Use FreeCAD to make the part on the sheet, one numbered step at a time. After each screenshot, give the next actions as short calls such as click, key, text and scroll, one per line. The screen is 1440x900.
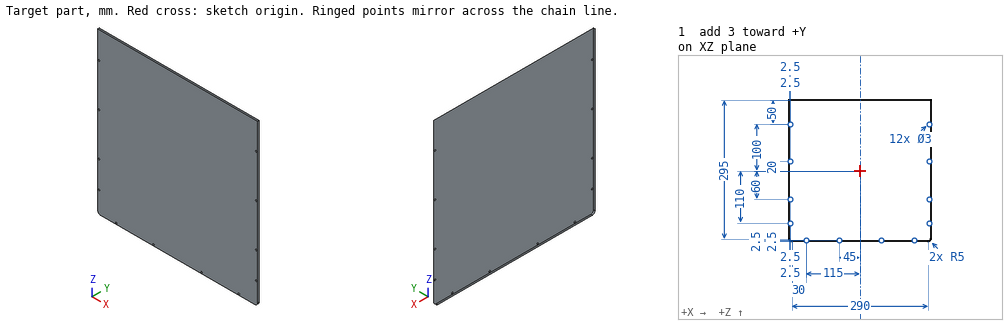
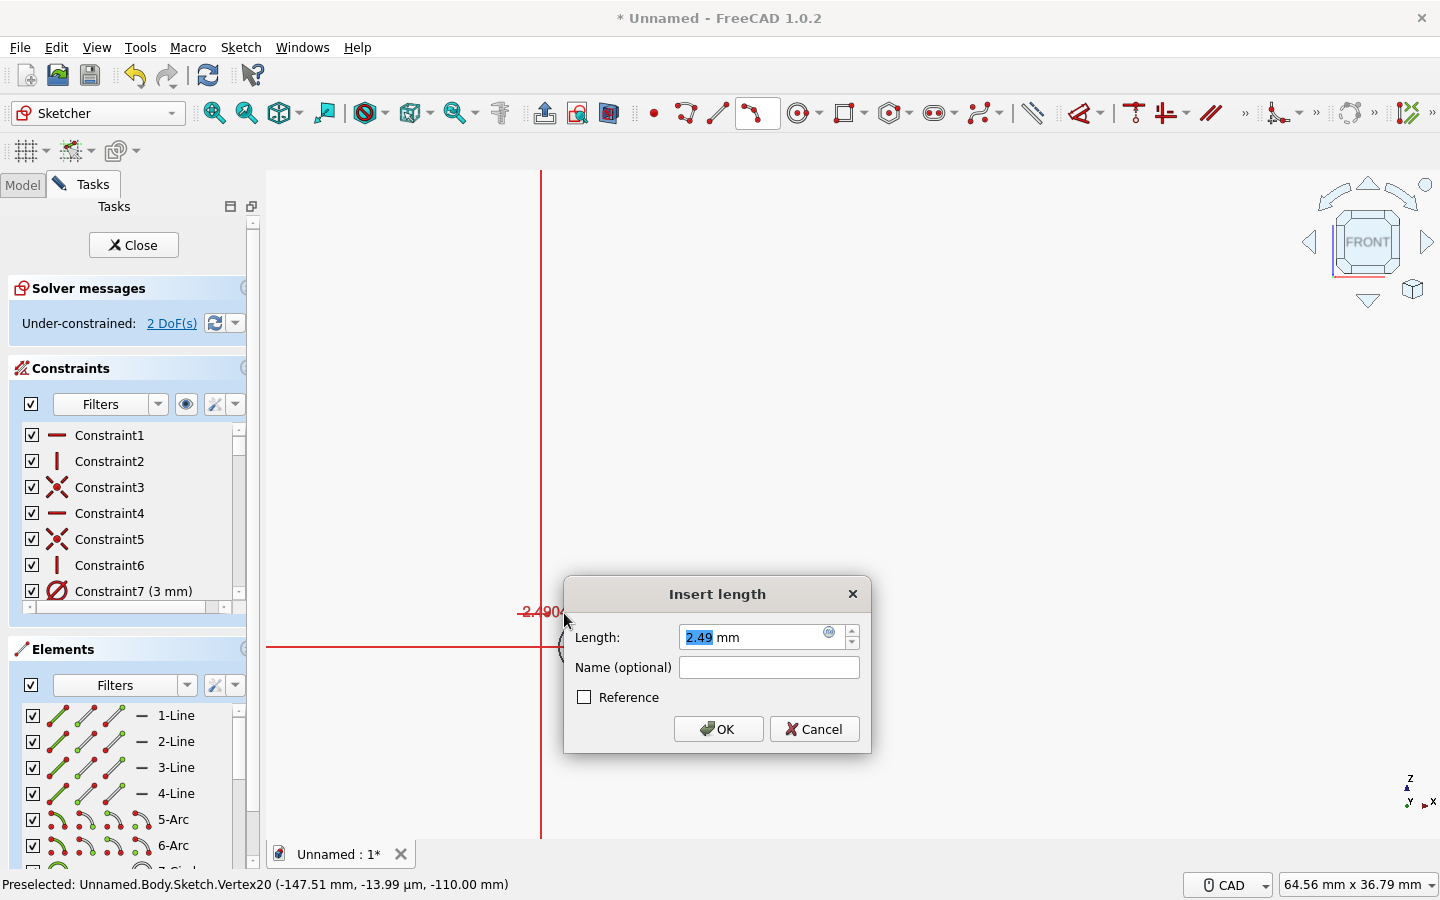
text(2.5)
key(Return)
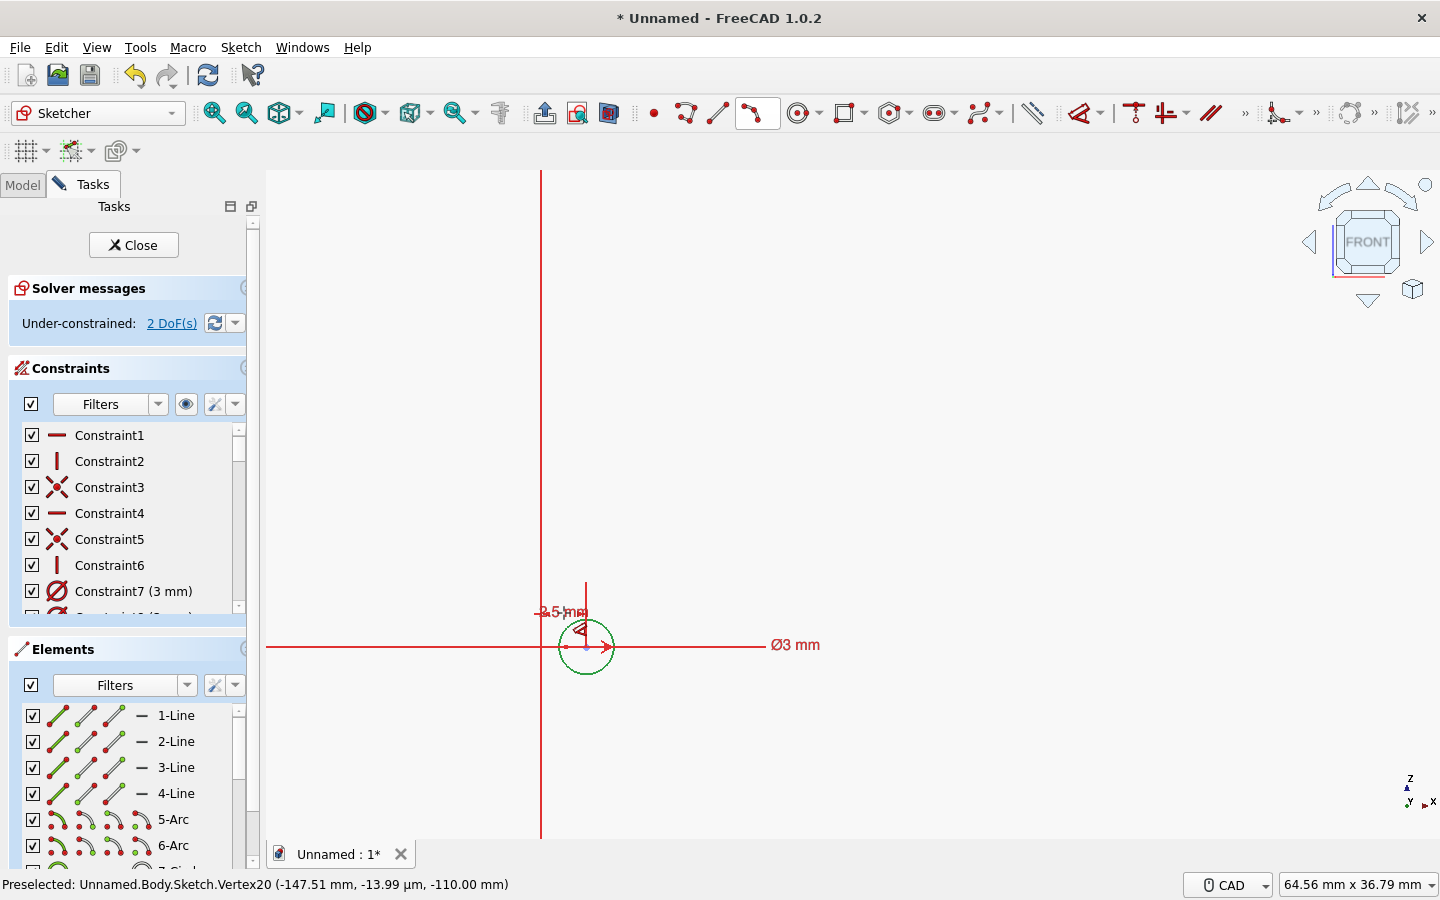
scroll(585, 654, down, 13)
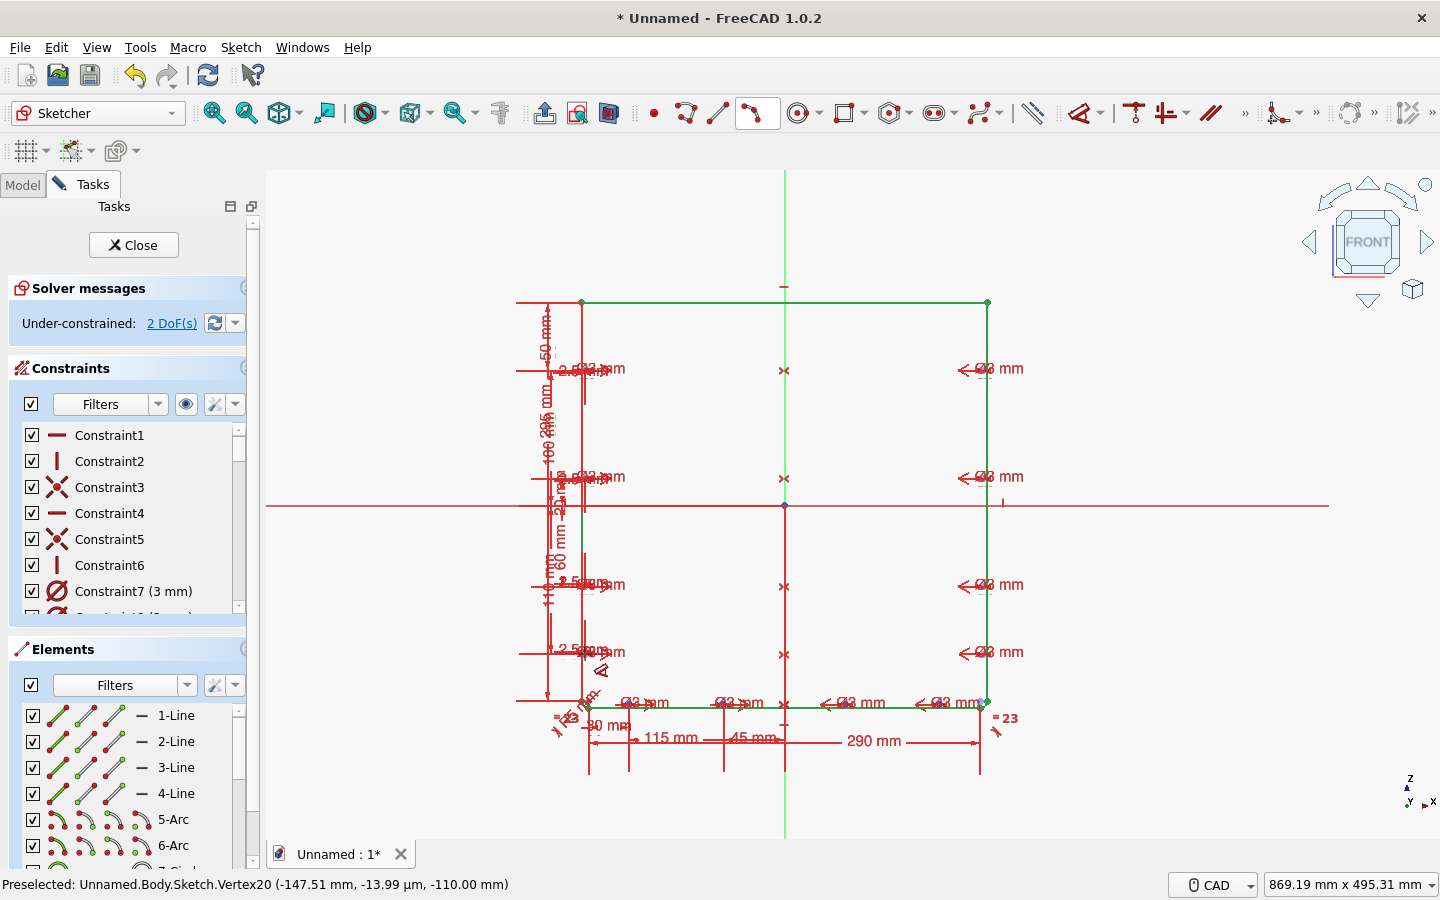
scroll(589, 708, up, 13)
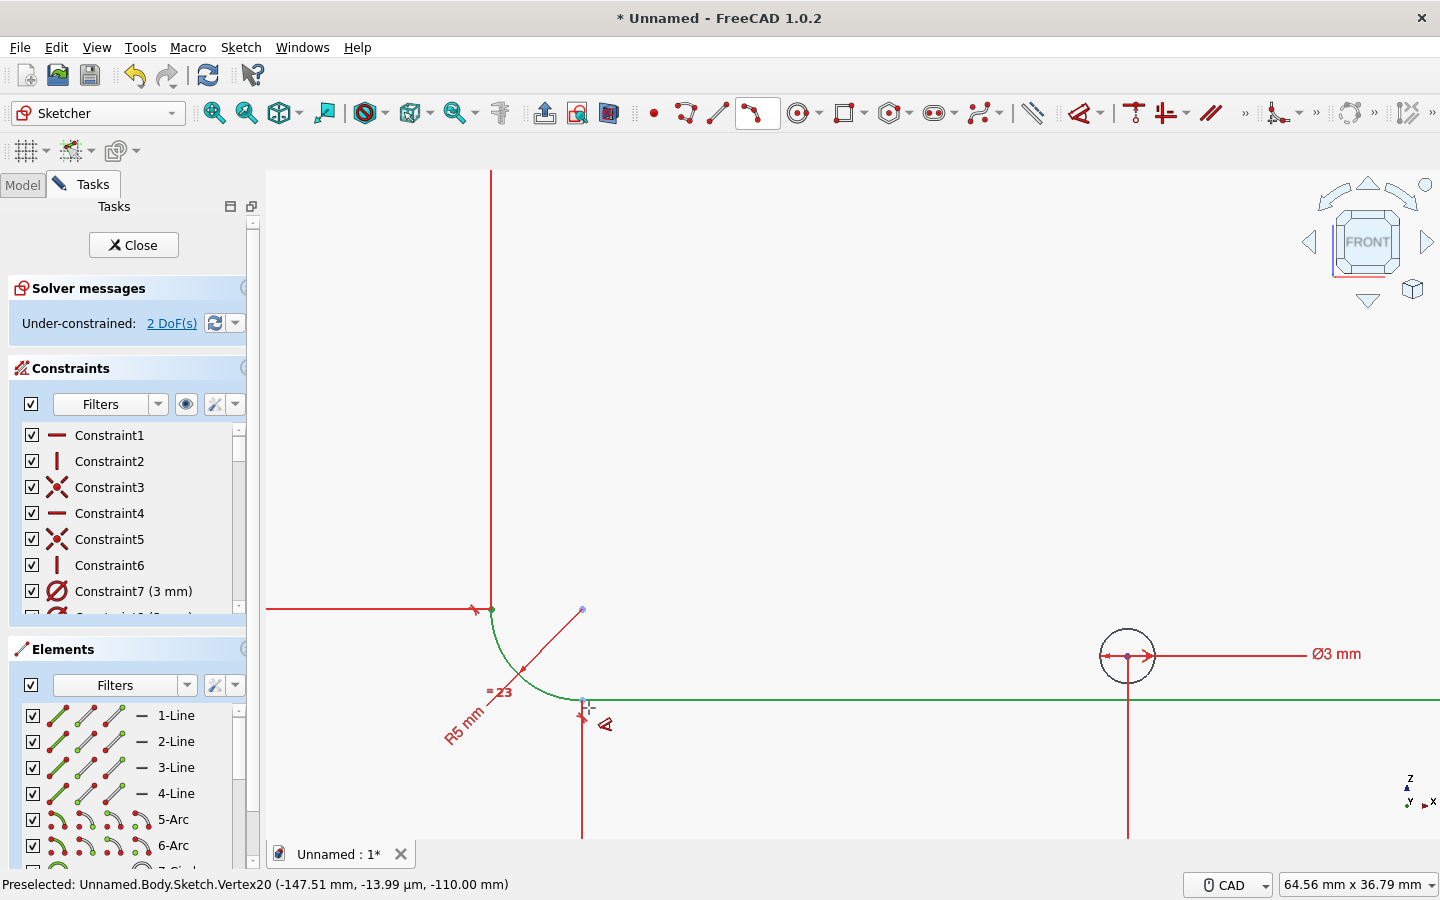
click(582, 700)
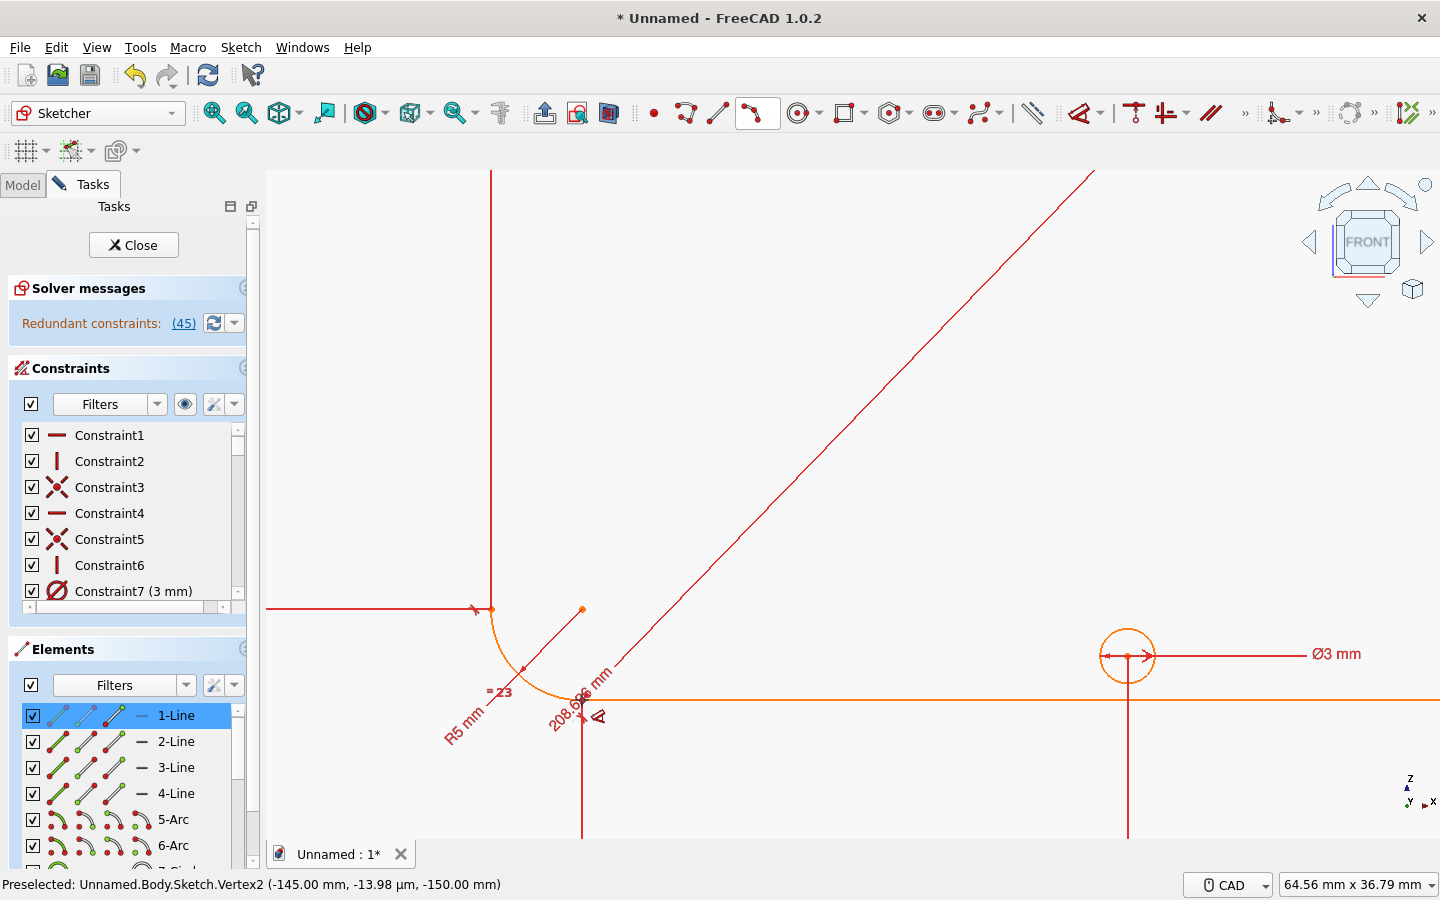
click(1128, 656)
click(548, 678)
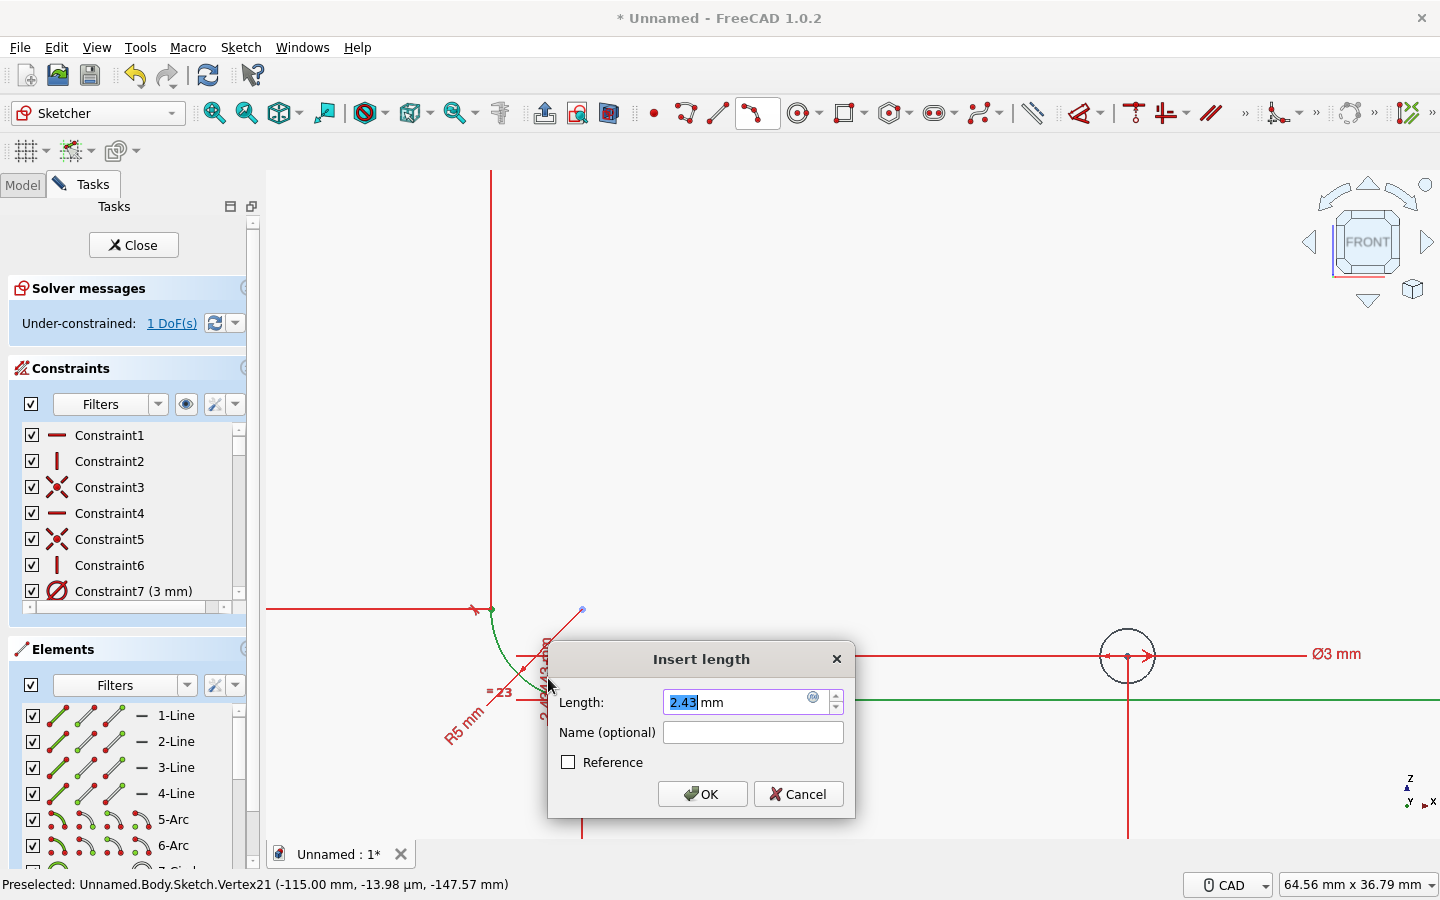
text(2.5)
key(Return)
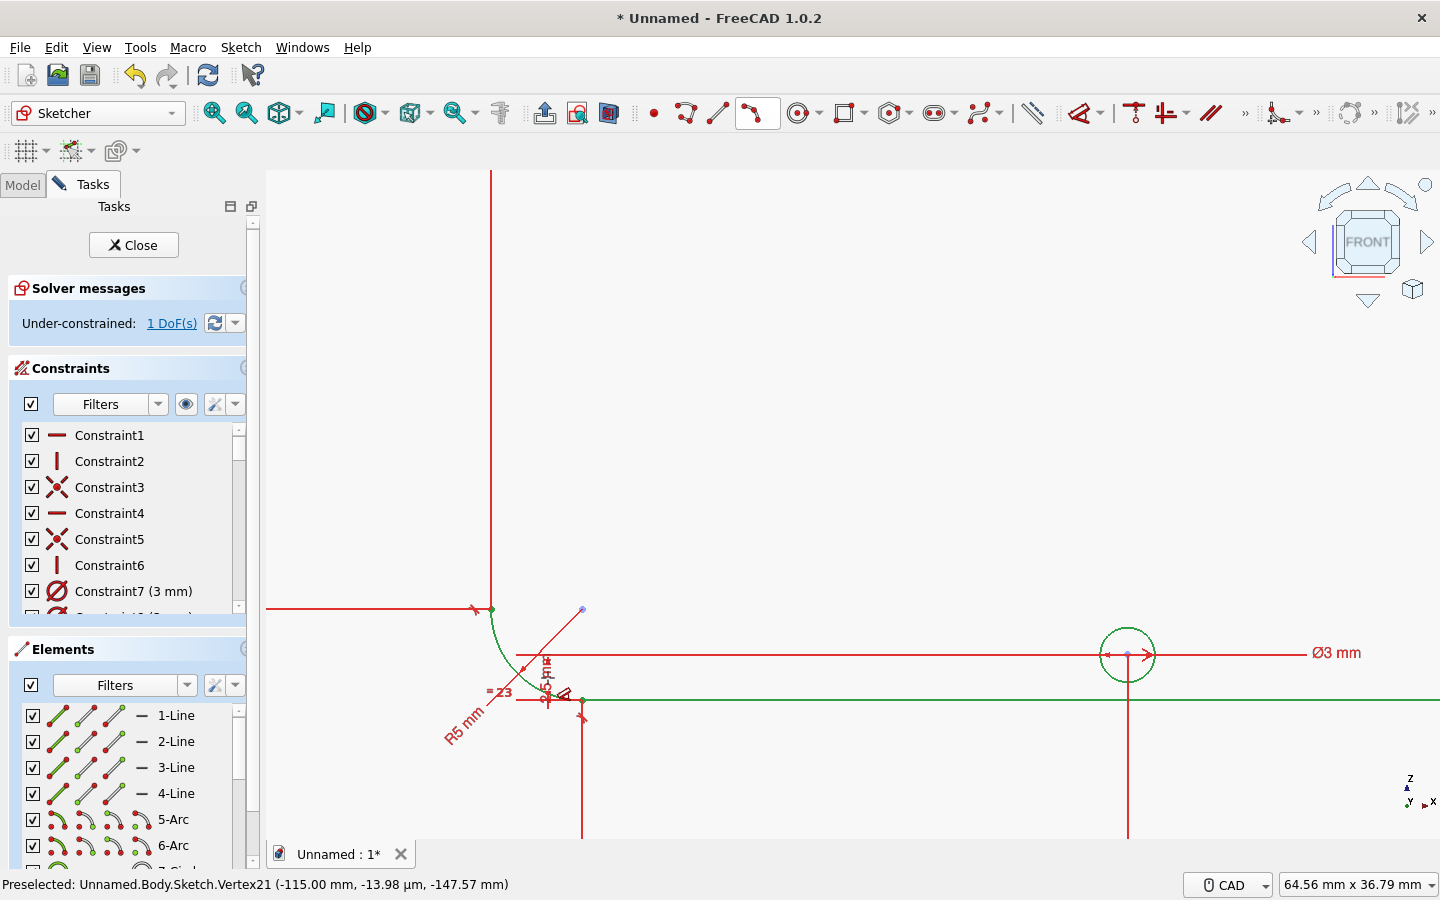
click(582, 700)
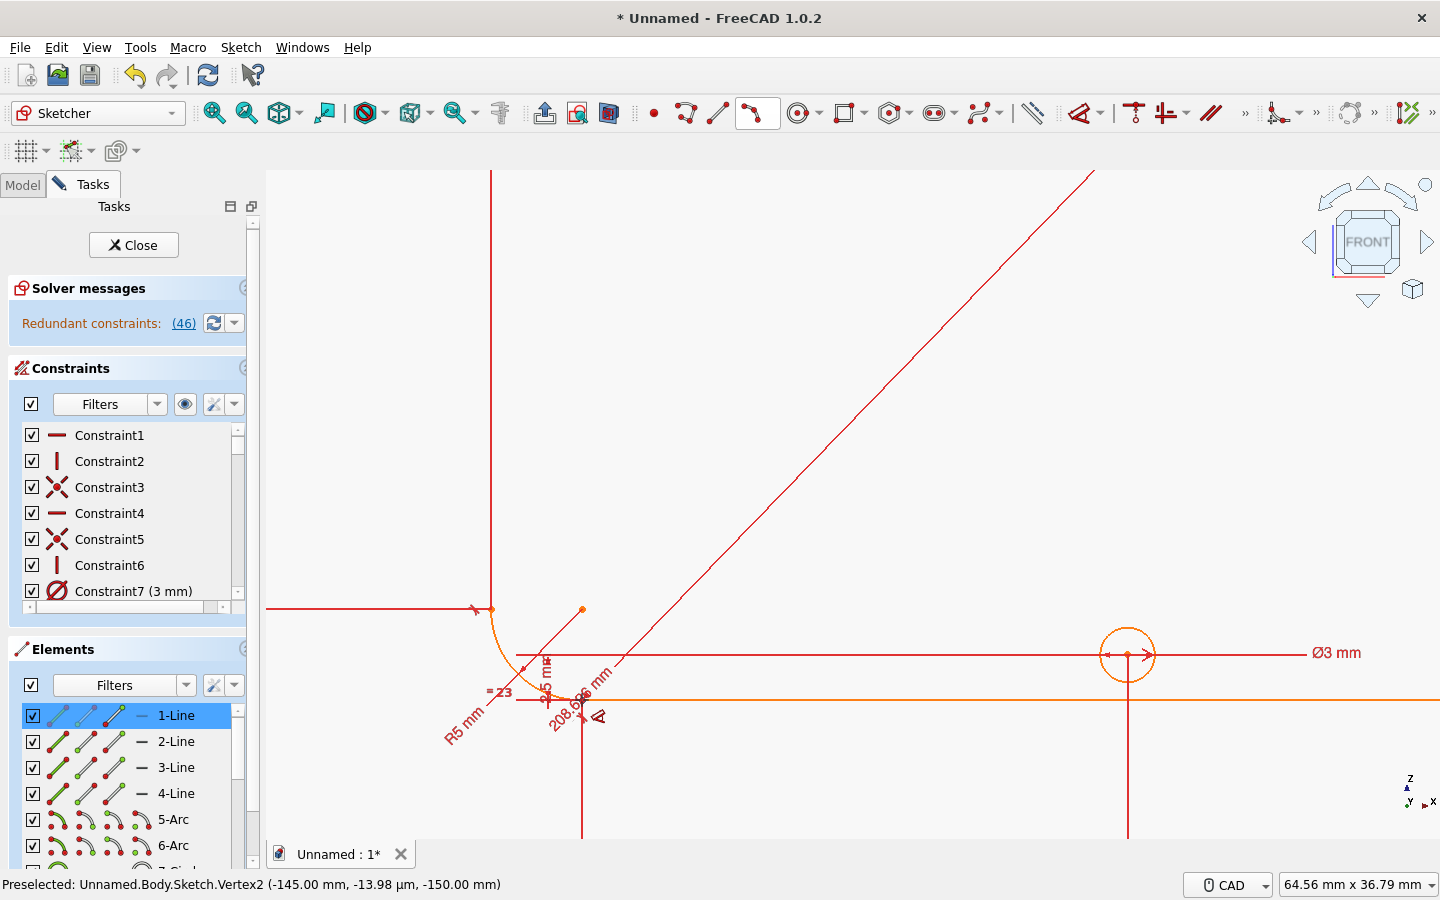
scroll(589, 708, down, 13)